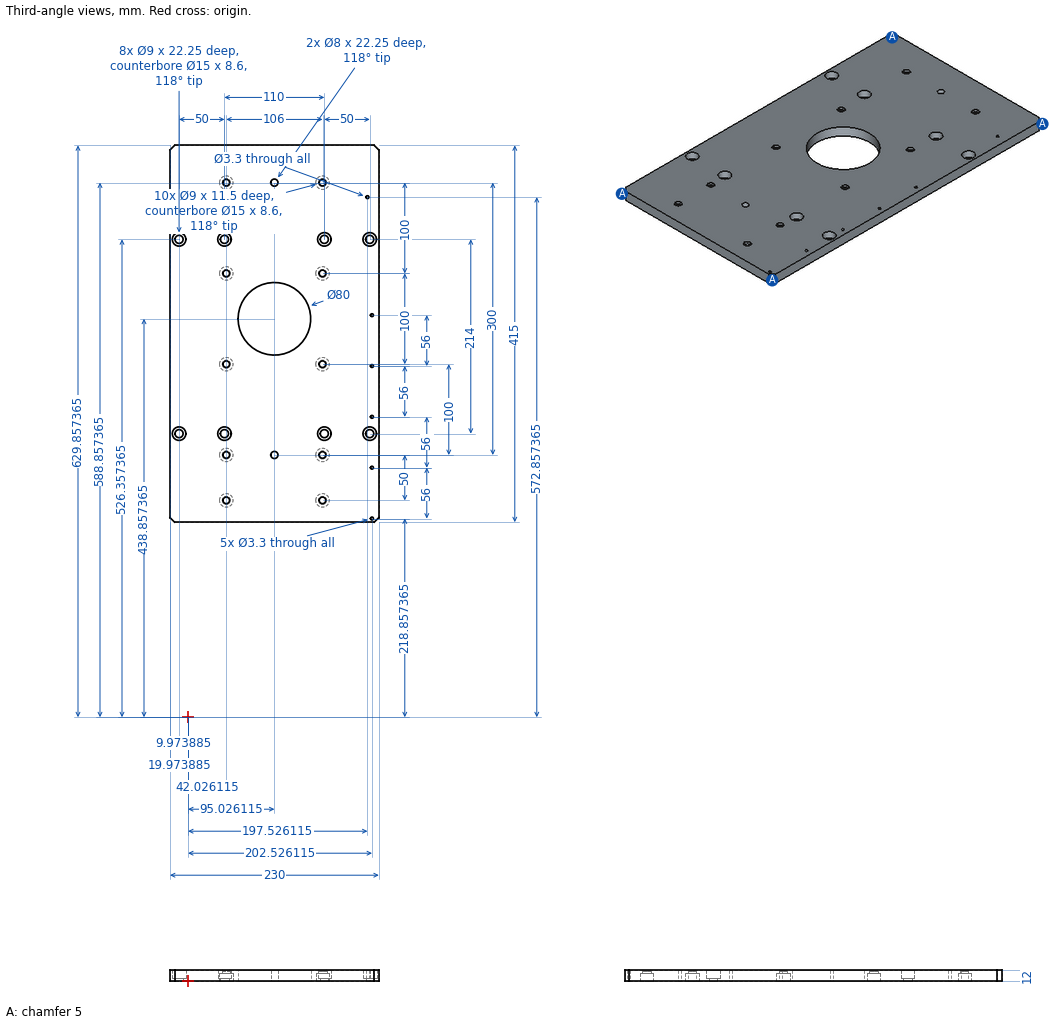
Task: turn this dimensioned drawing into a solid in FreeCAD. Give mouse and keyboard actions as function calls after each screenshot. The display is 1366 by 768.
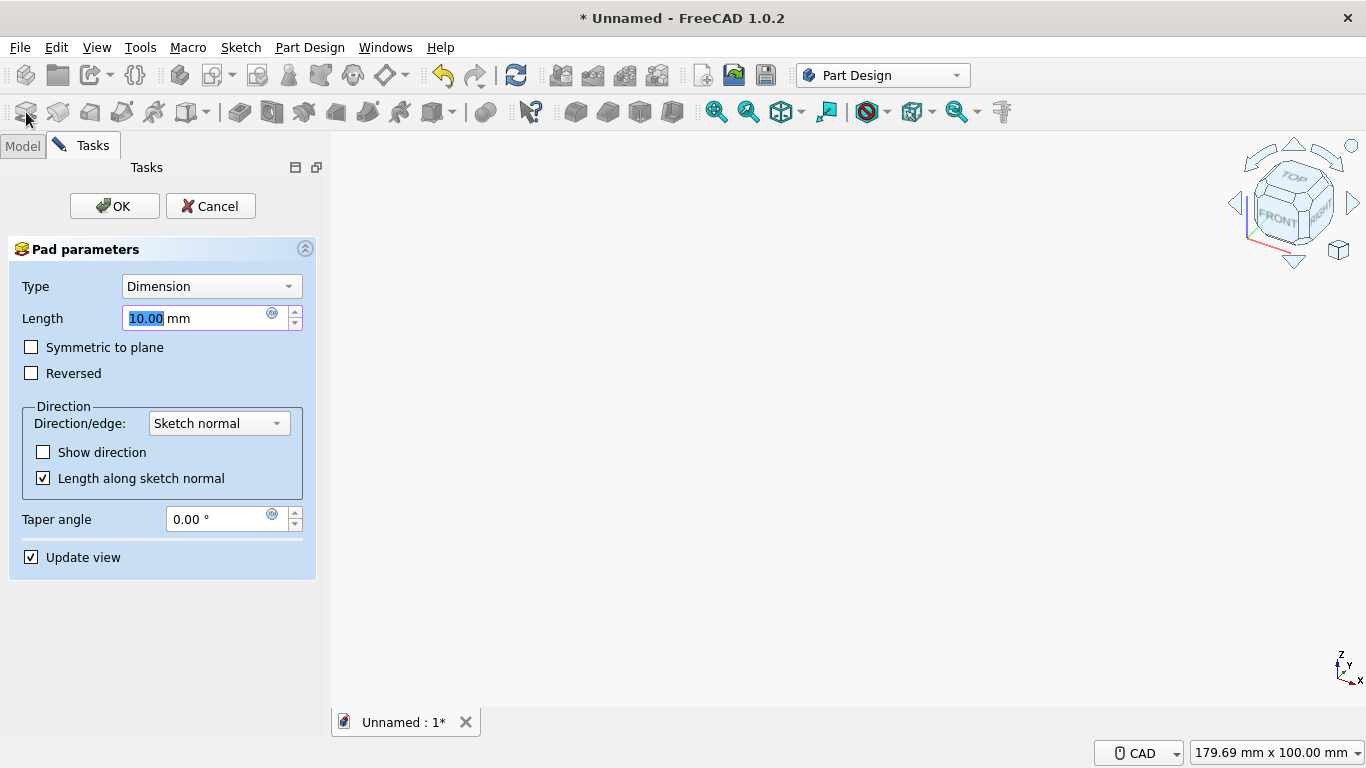
text(12)
key(Tab)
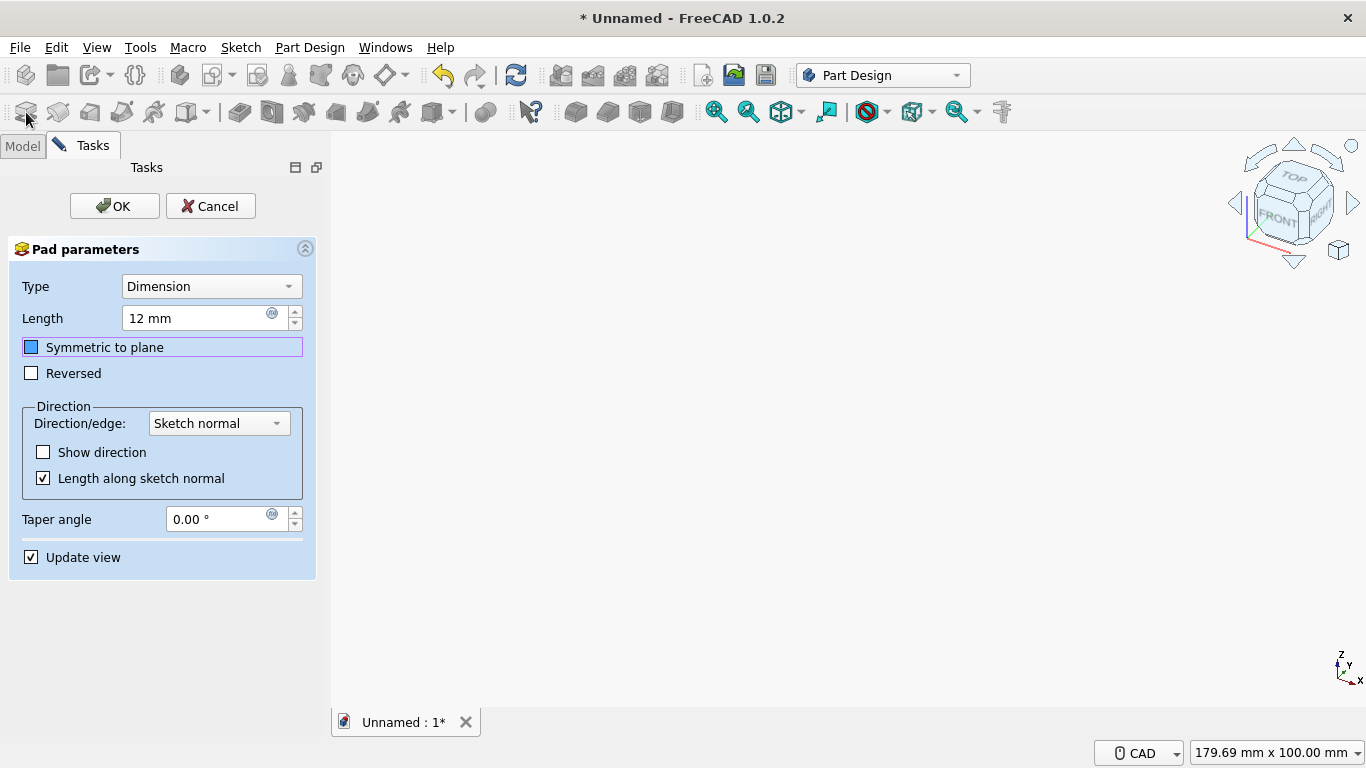
click(115, 206)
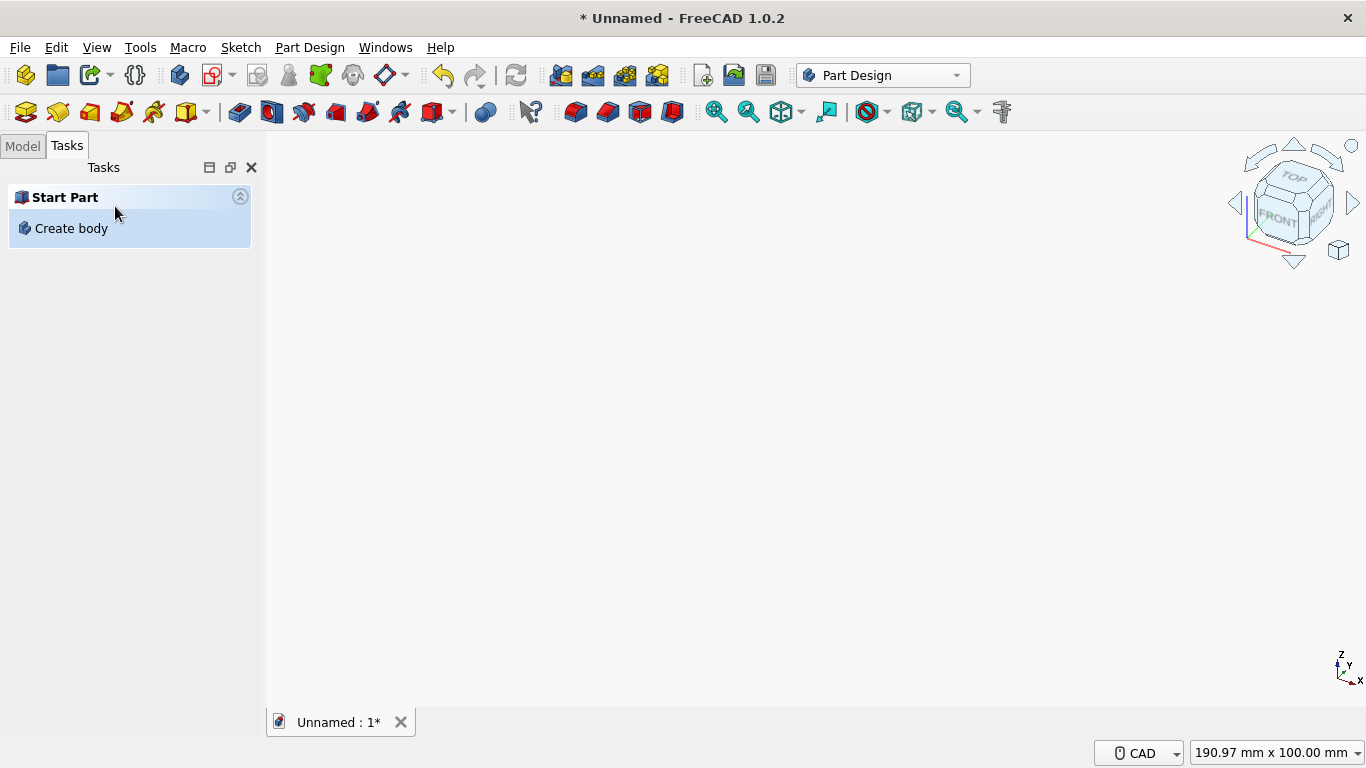
click(718, 112)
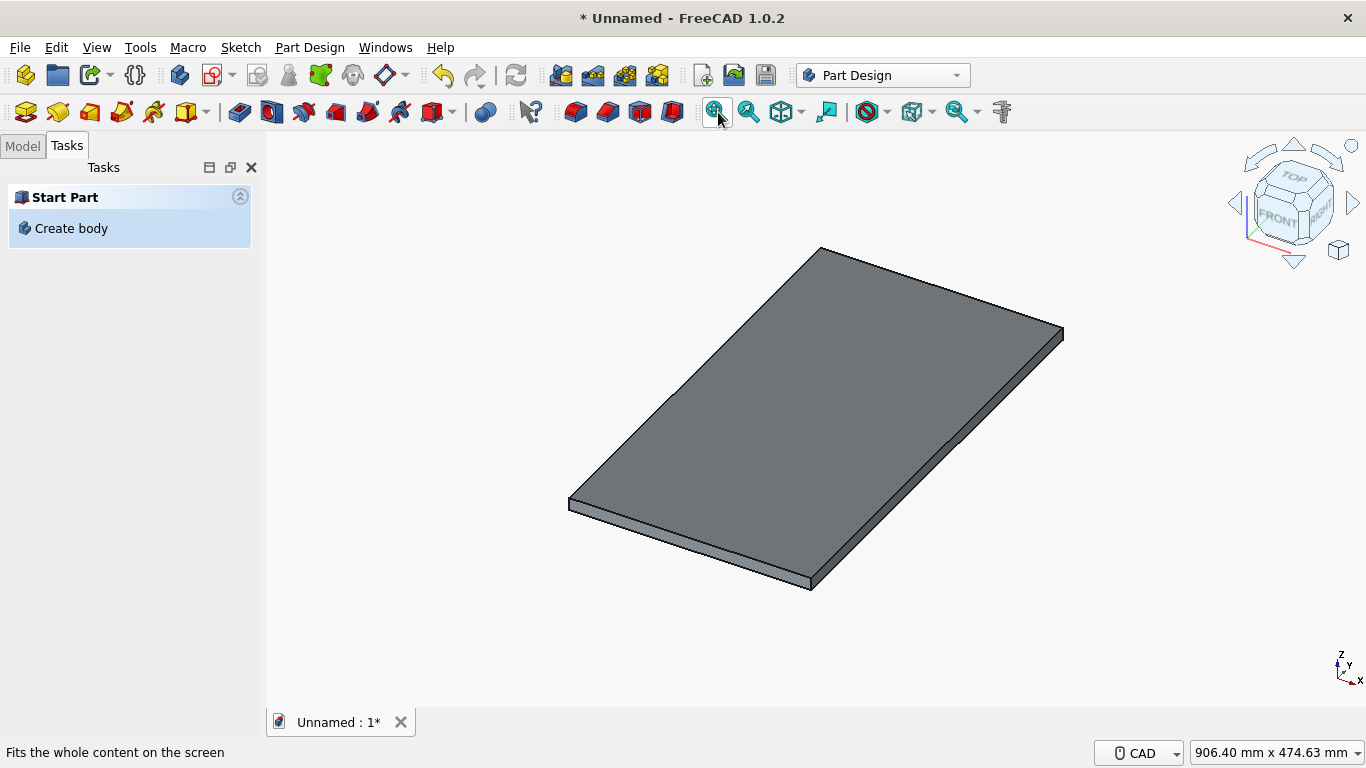
click(811, 584)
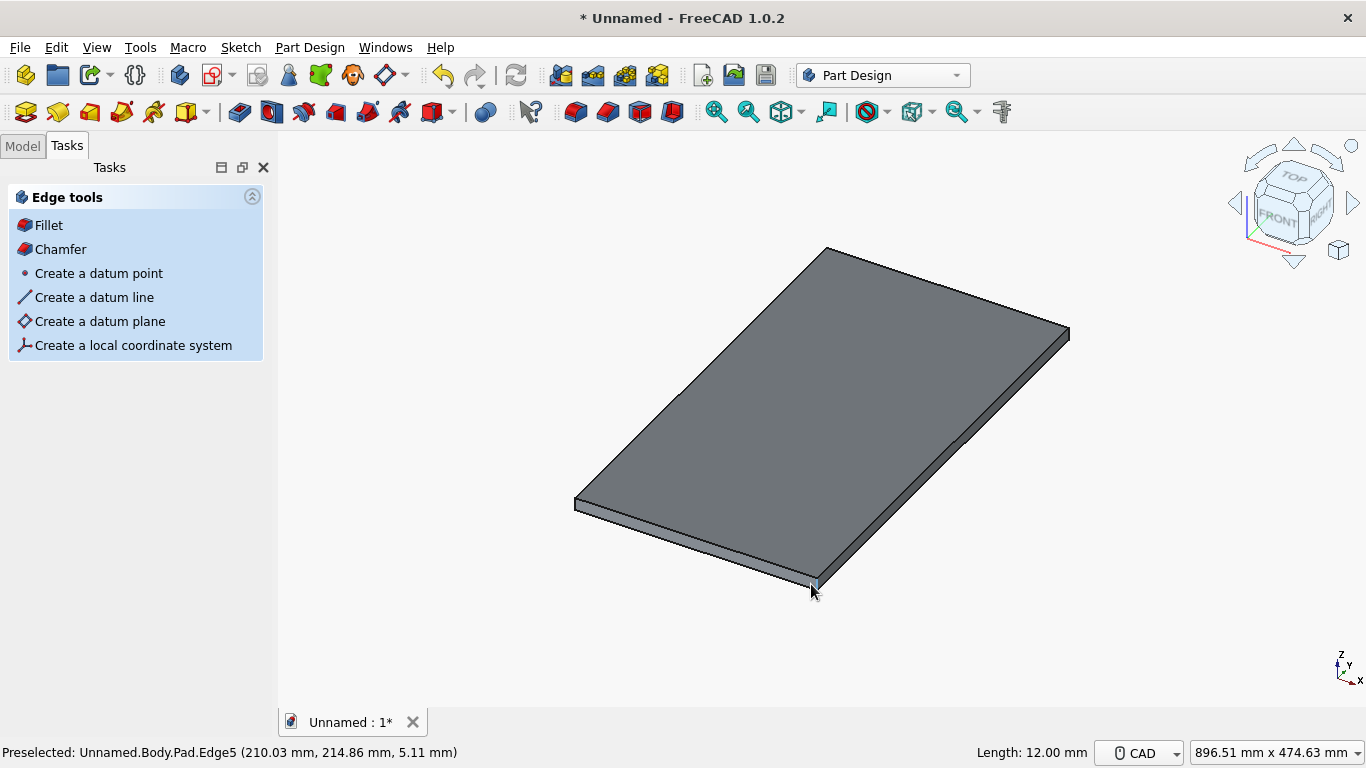
scroll(575, 503, up, 6)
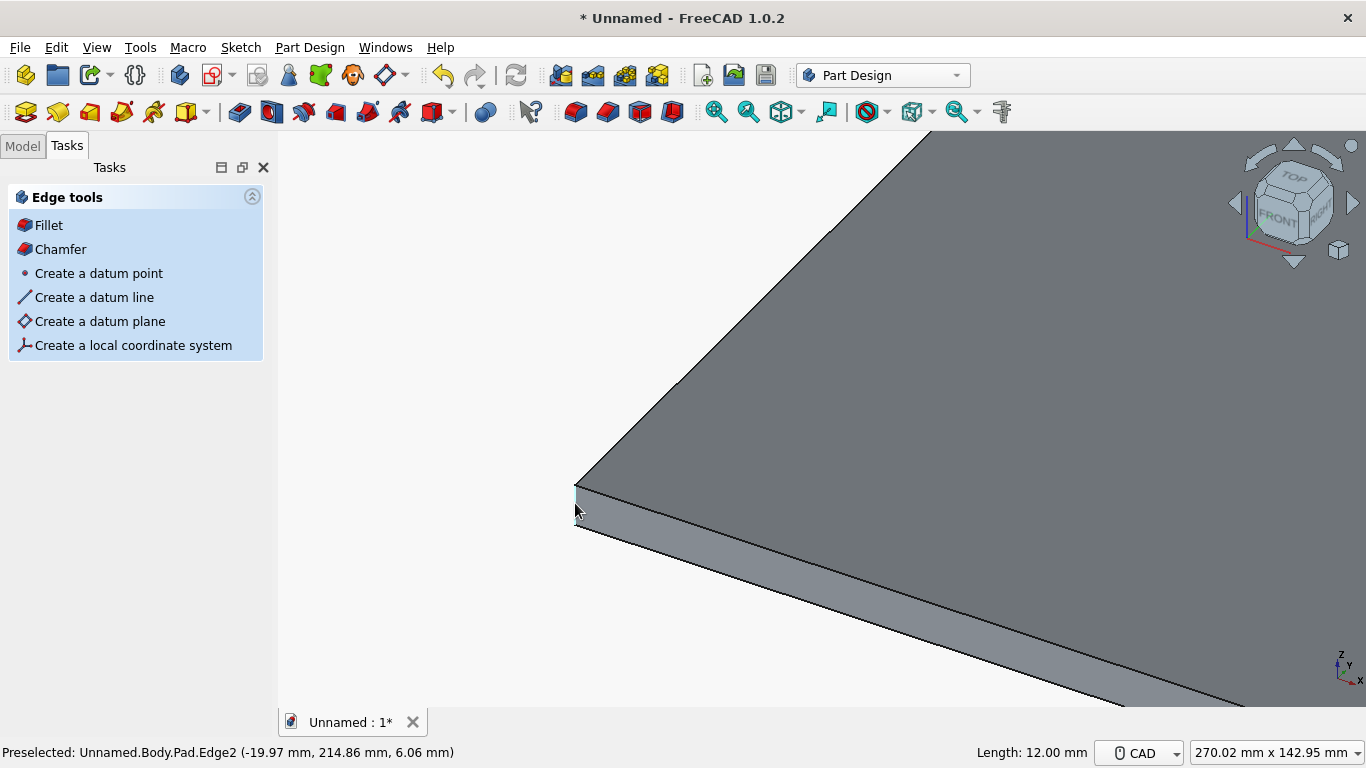
click(718, 112)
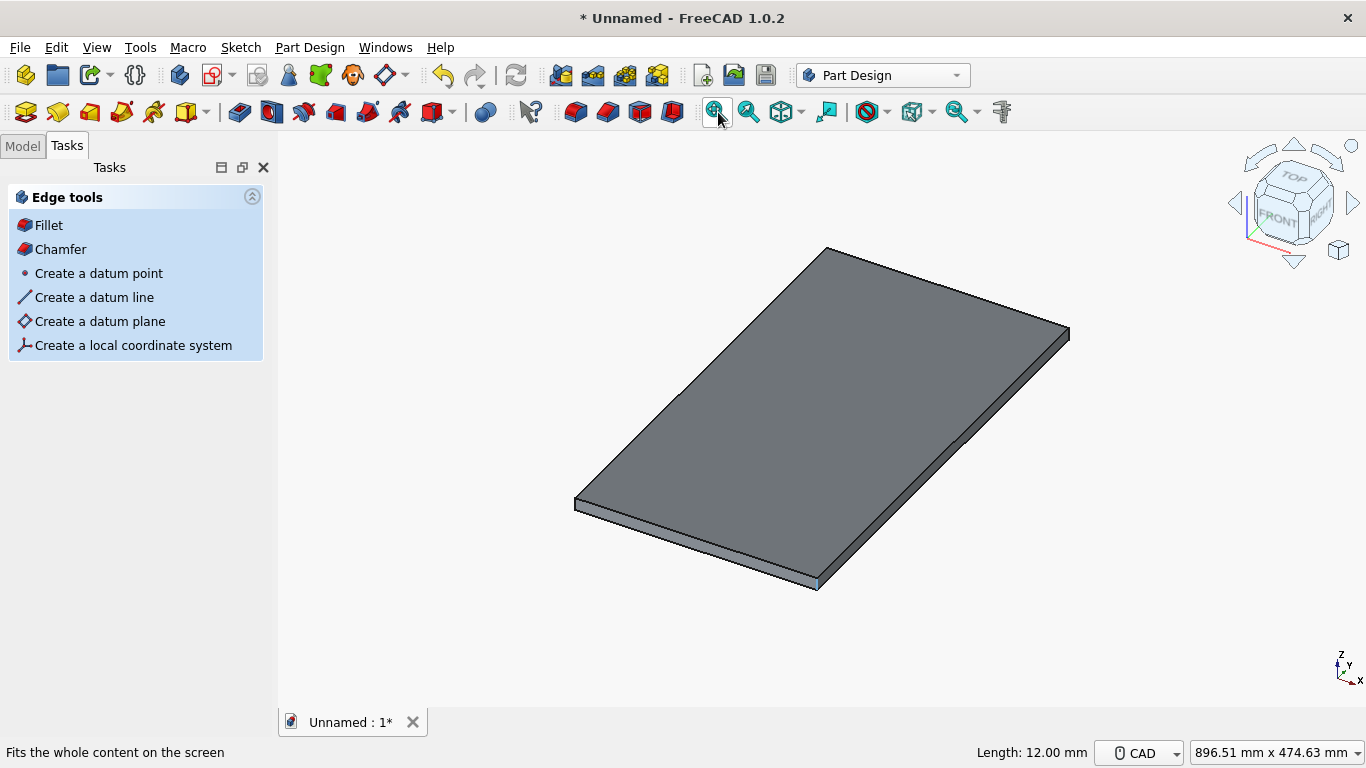
key(0)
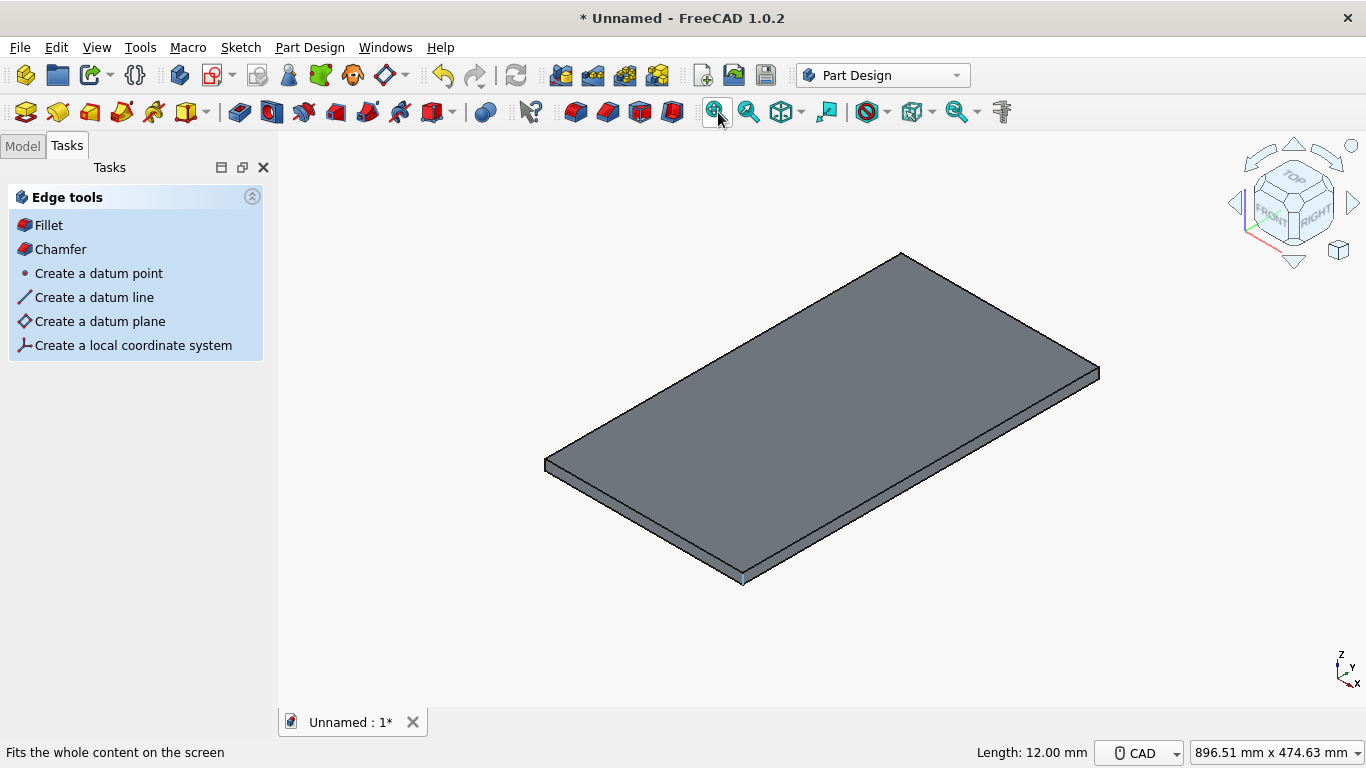
scroll(545, 464, up, 6)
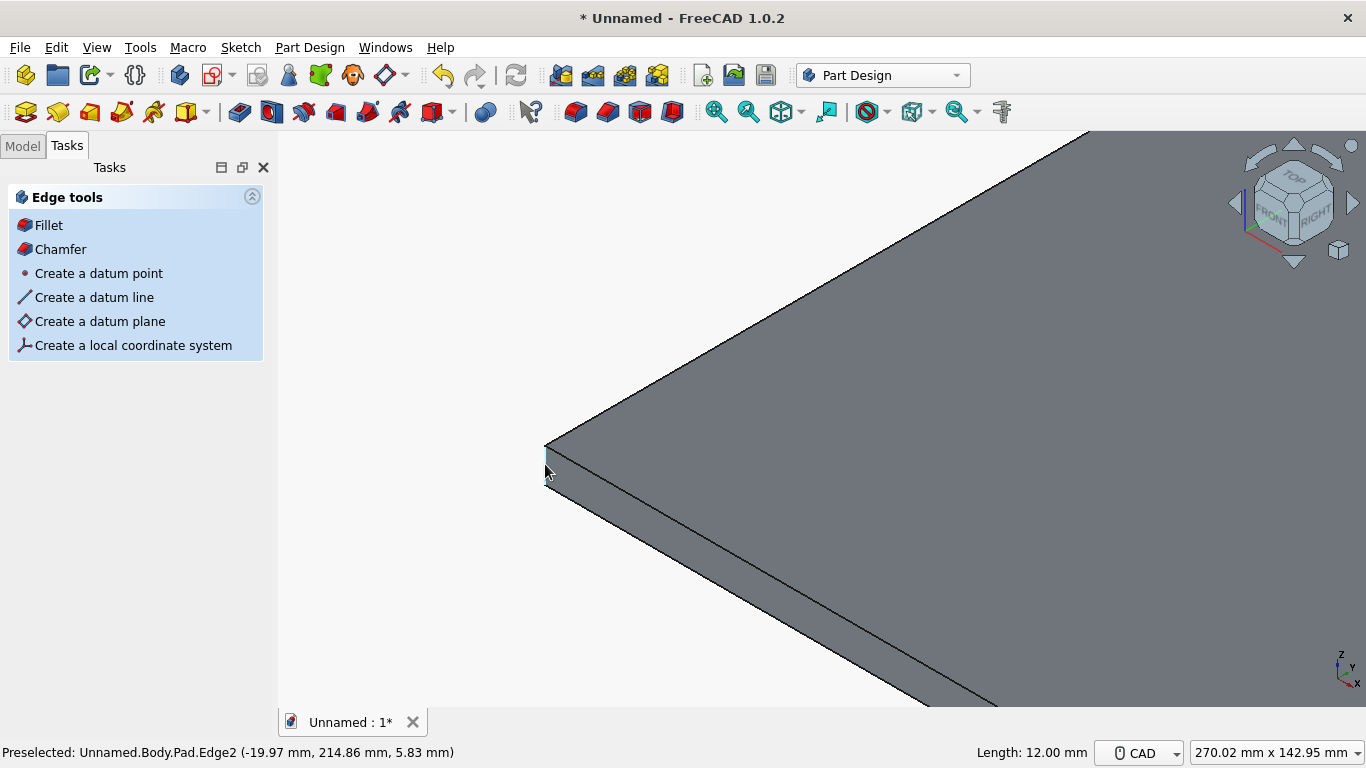
click(718, 112)